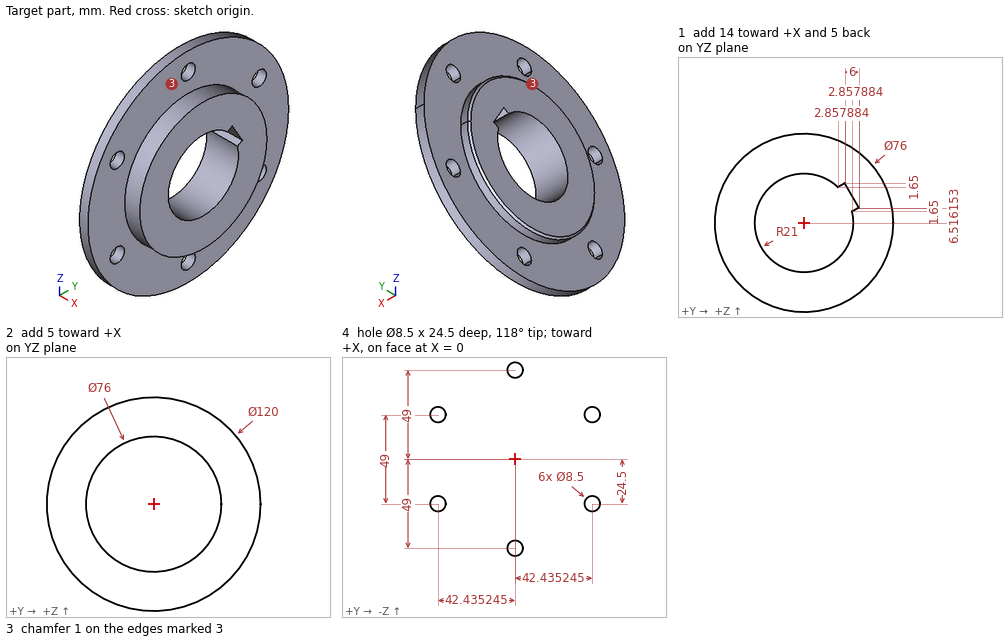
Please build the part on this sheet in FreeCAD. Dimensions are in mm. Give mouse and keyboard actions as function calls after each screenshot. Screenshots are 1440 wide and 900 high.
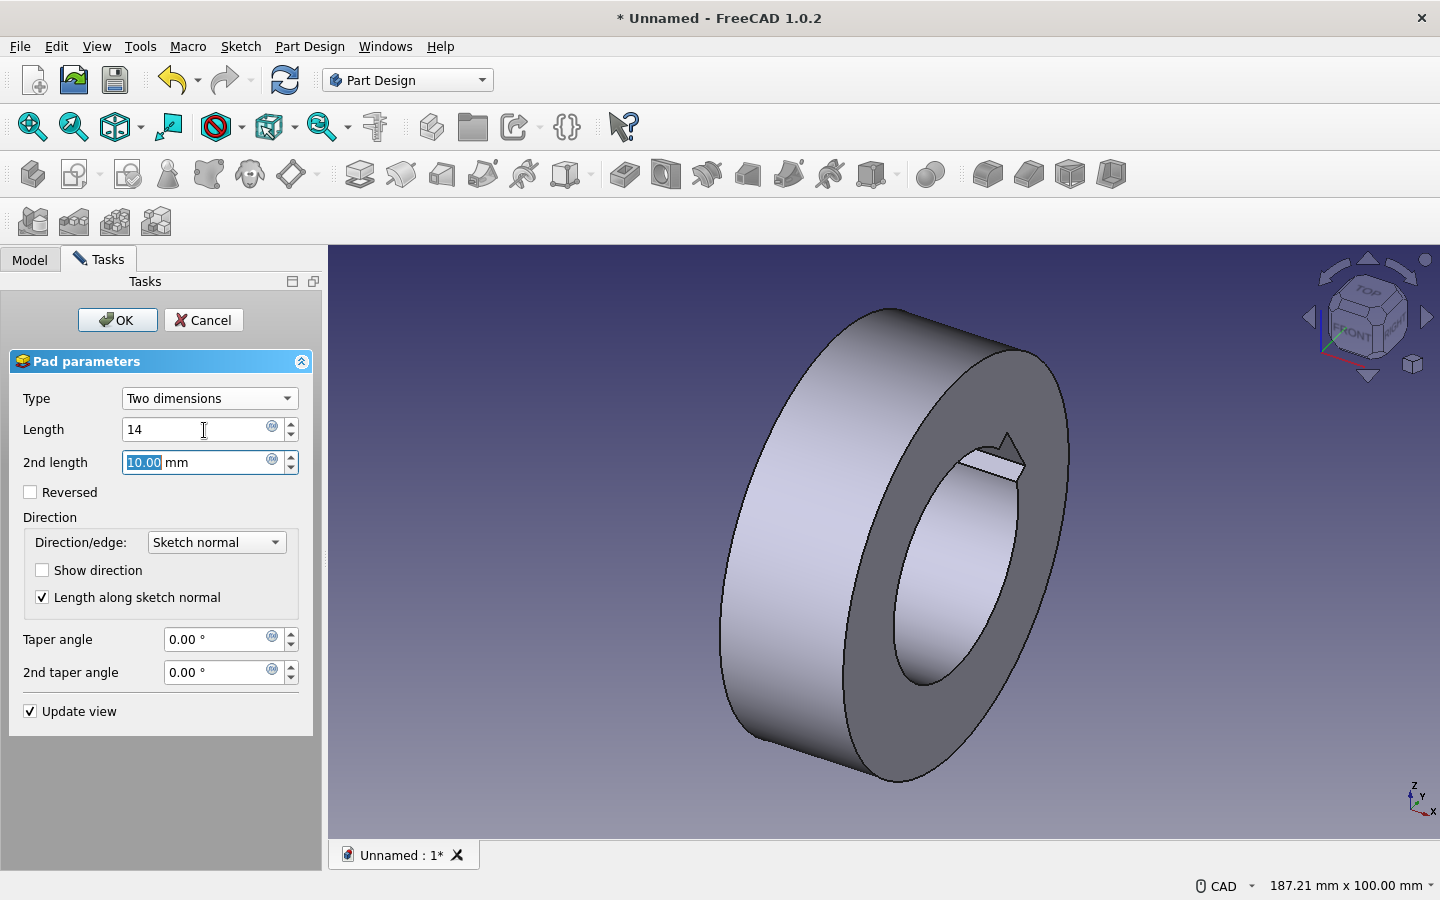
text(5)
key(Tab)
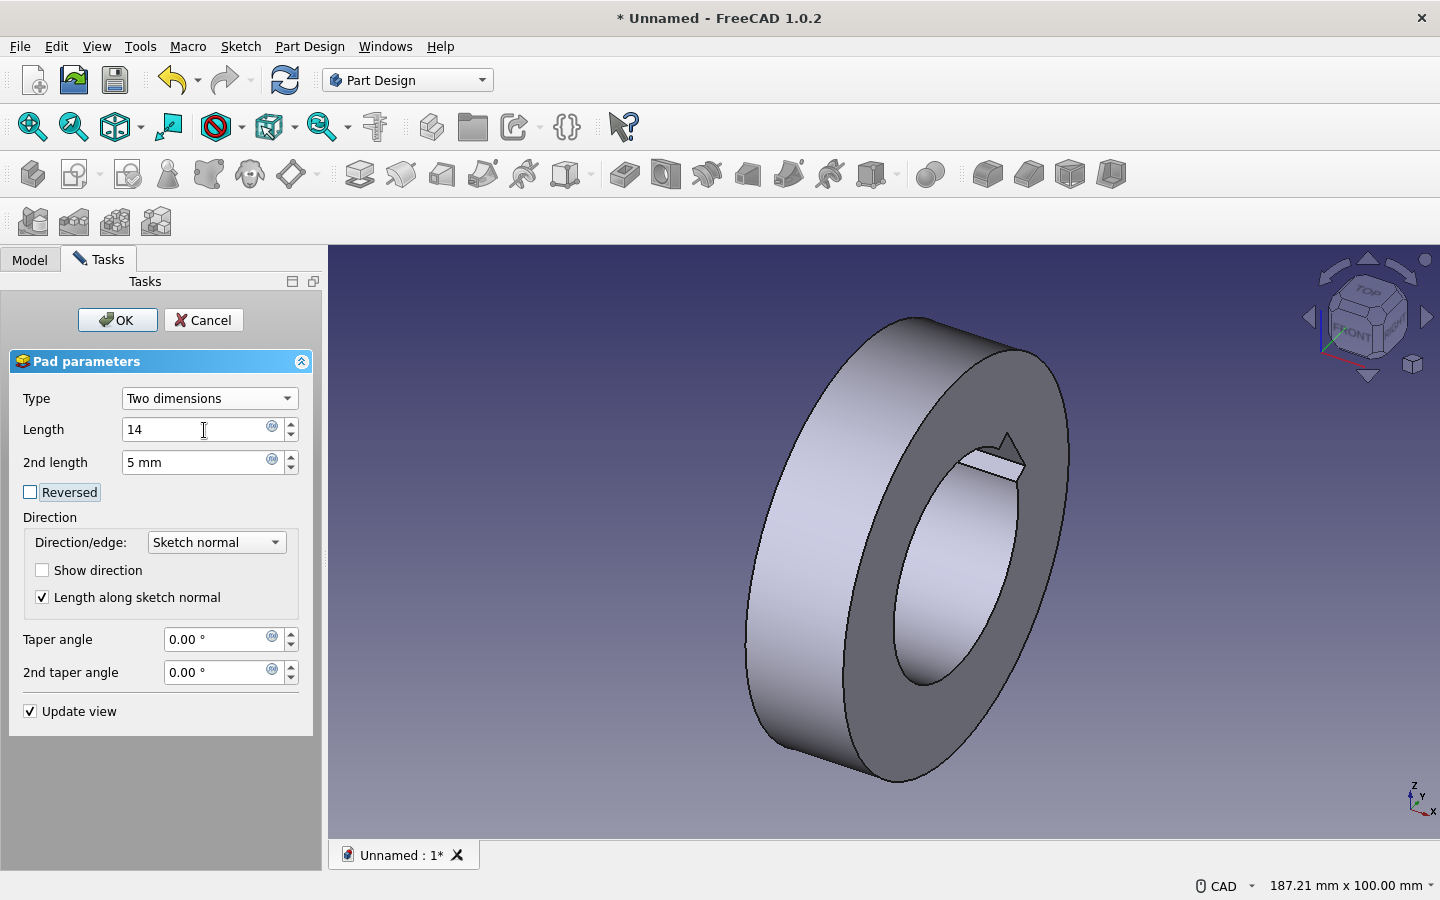
click(118, 320)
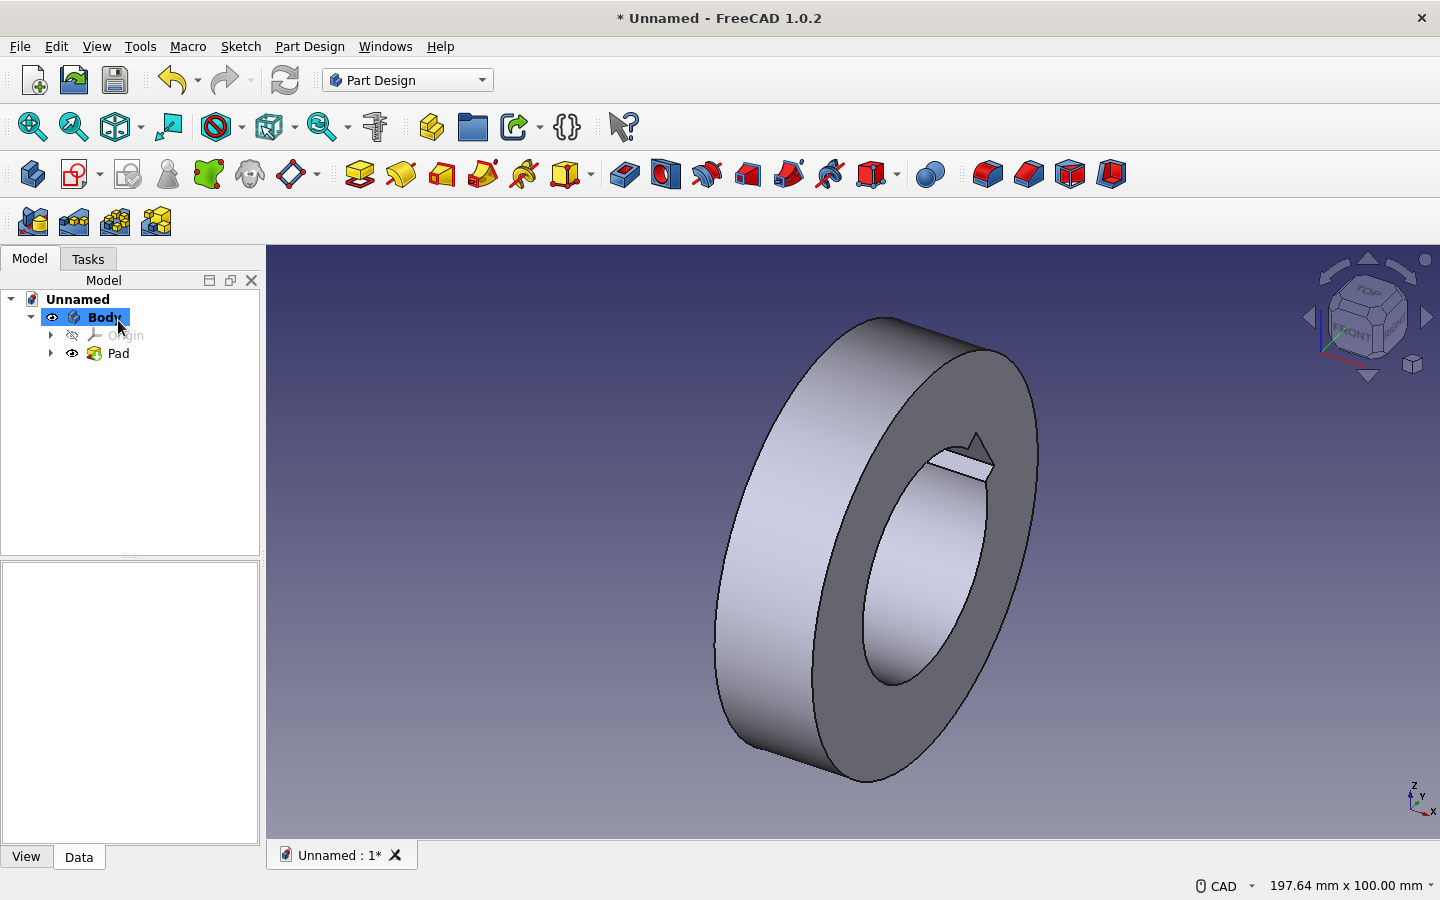
click(33, 128)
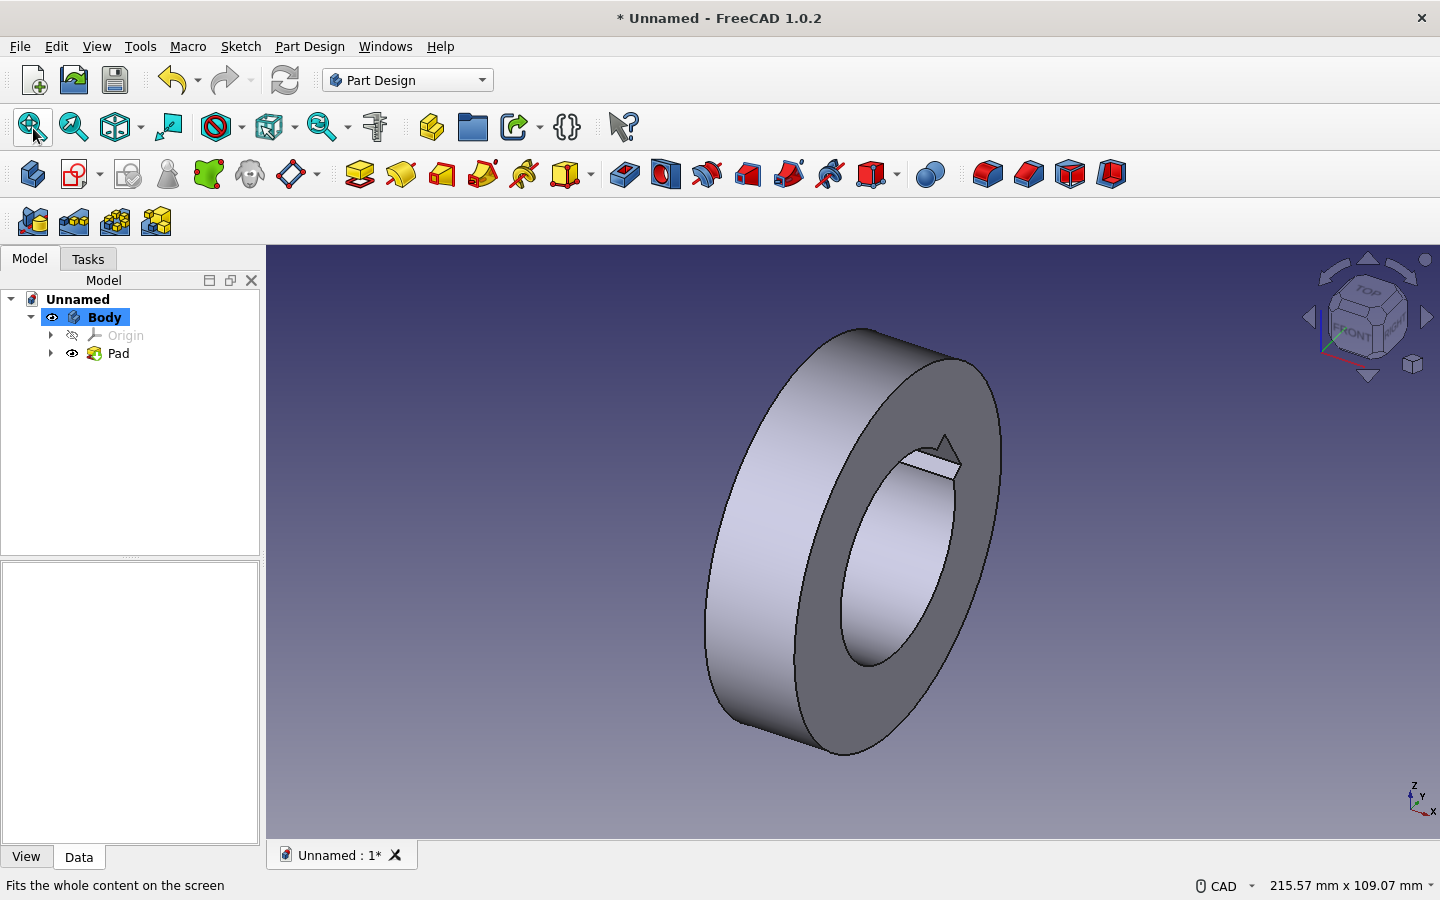
click(74, 174)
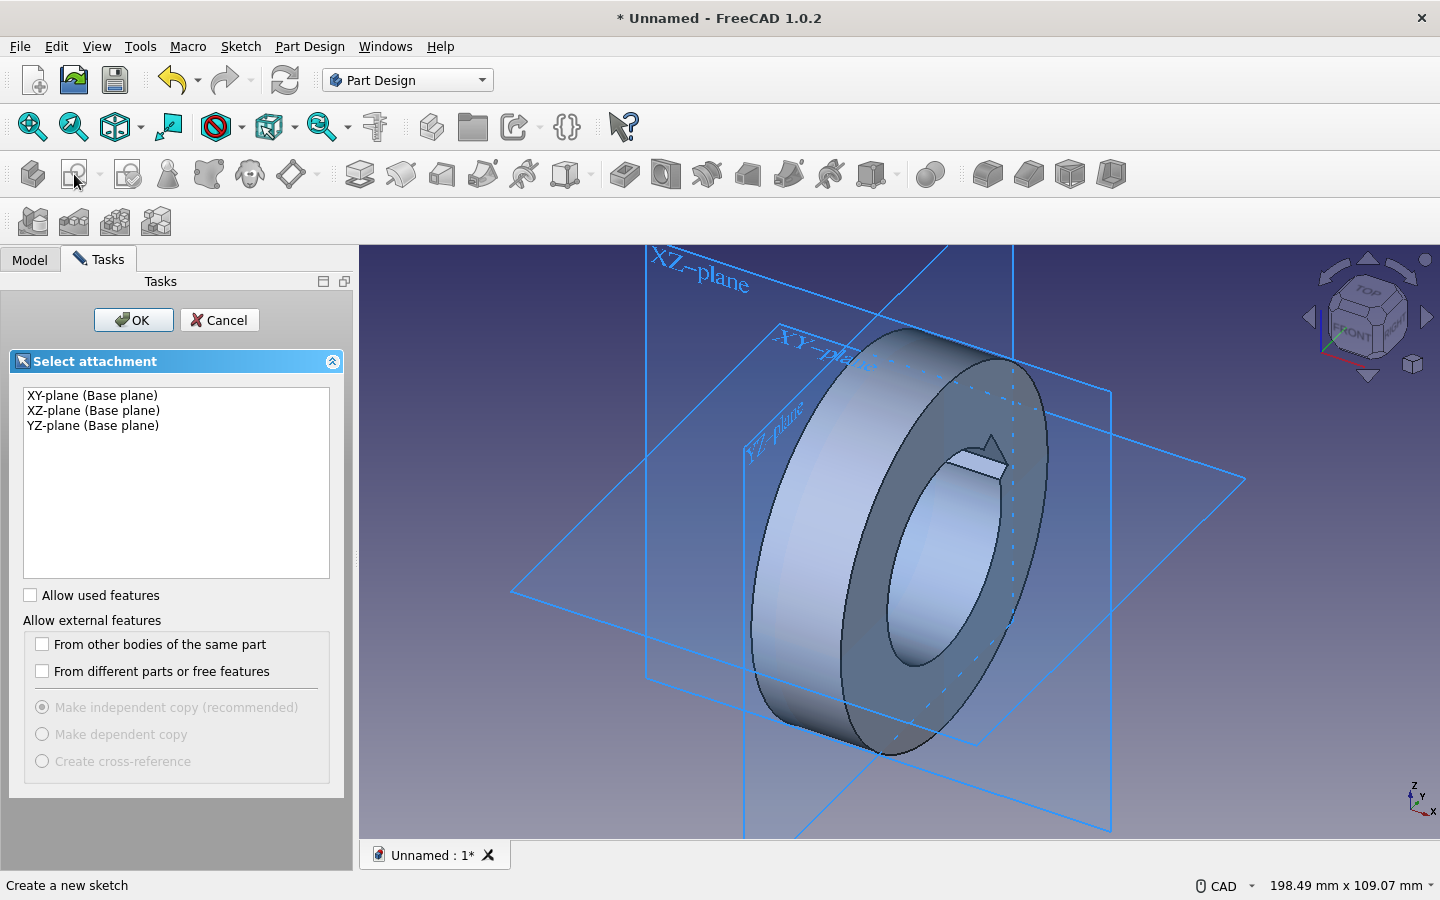
click(84, 426)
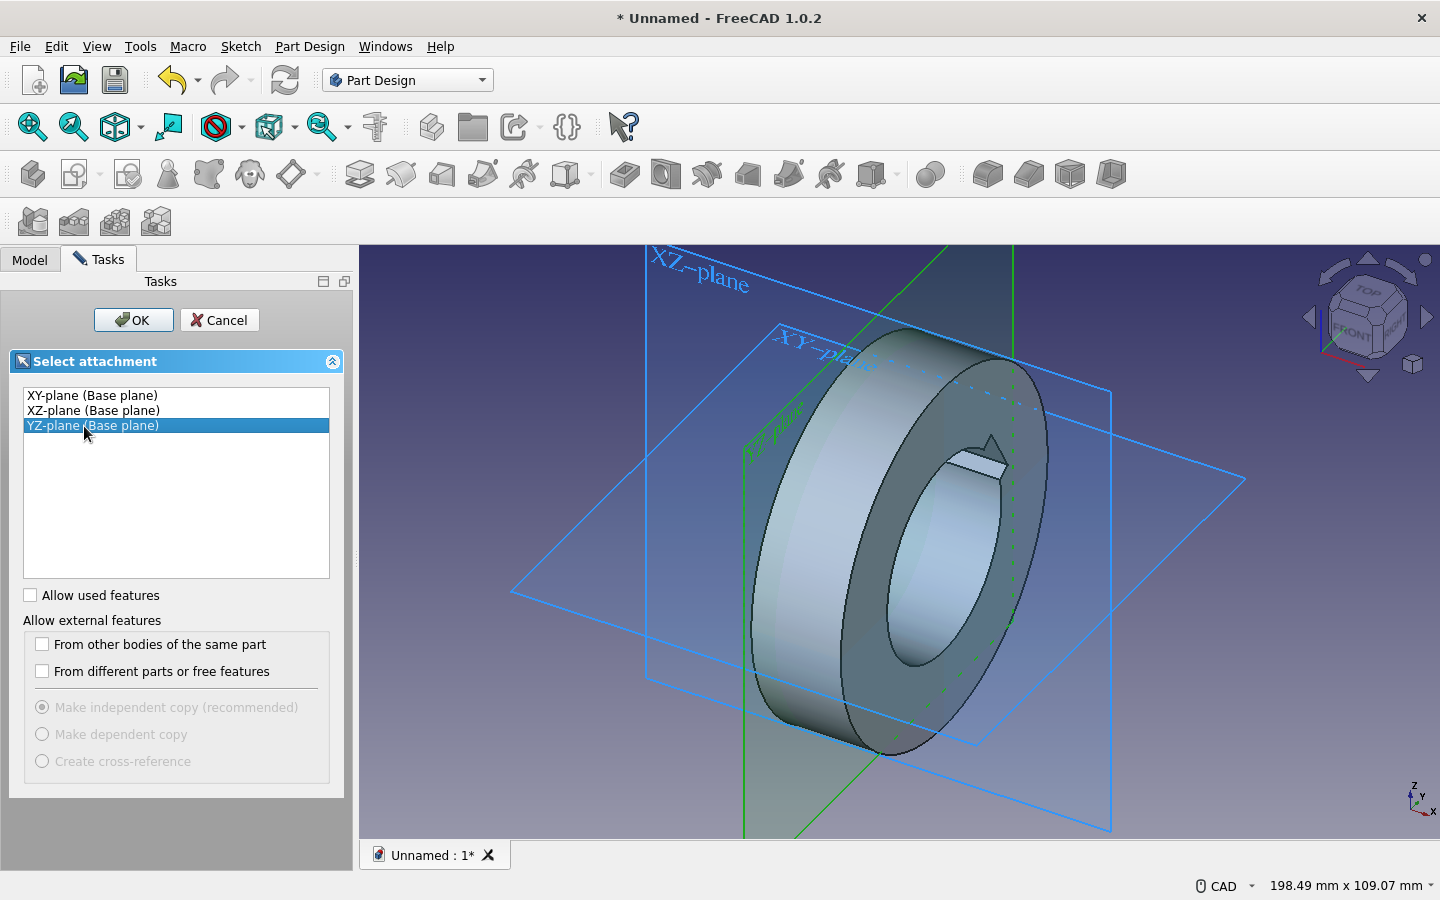
click(134, 320)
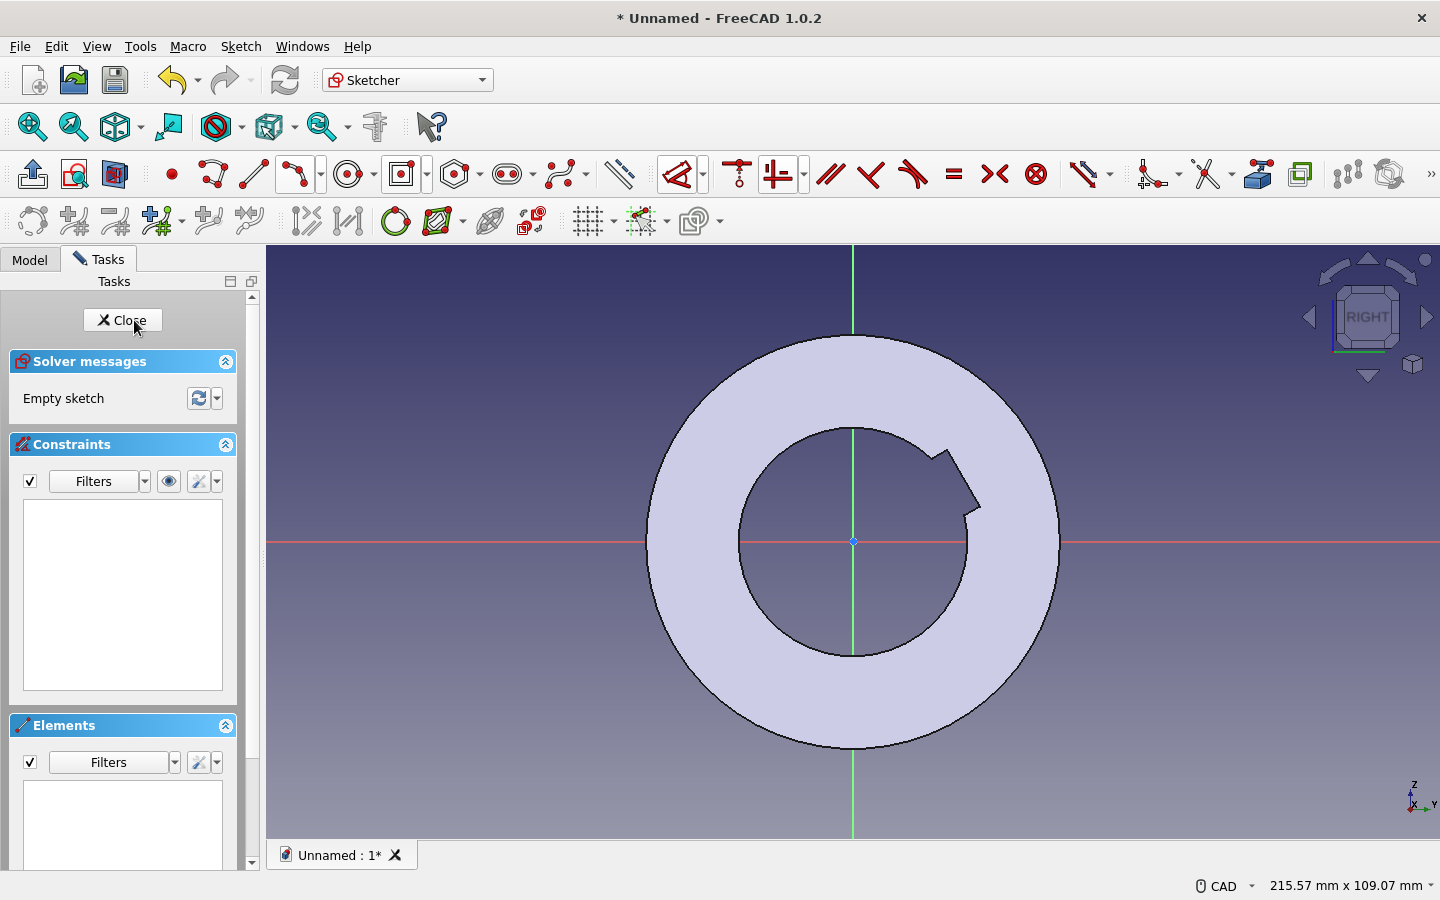
click(115, 174)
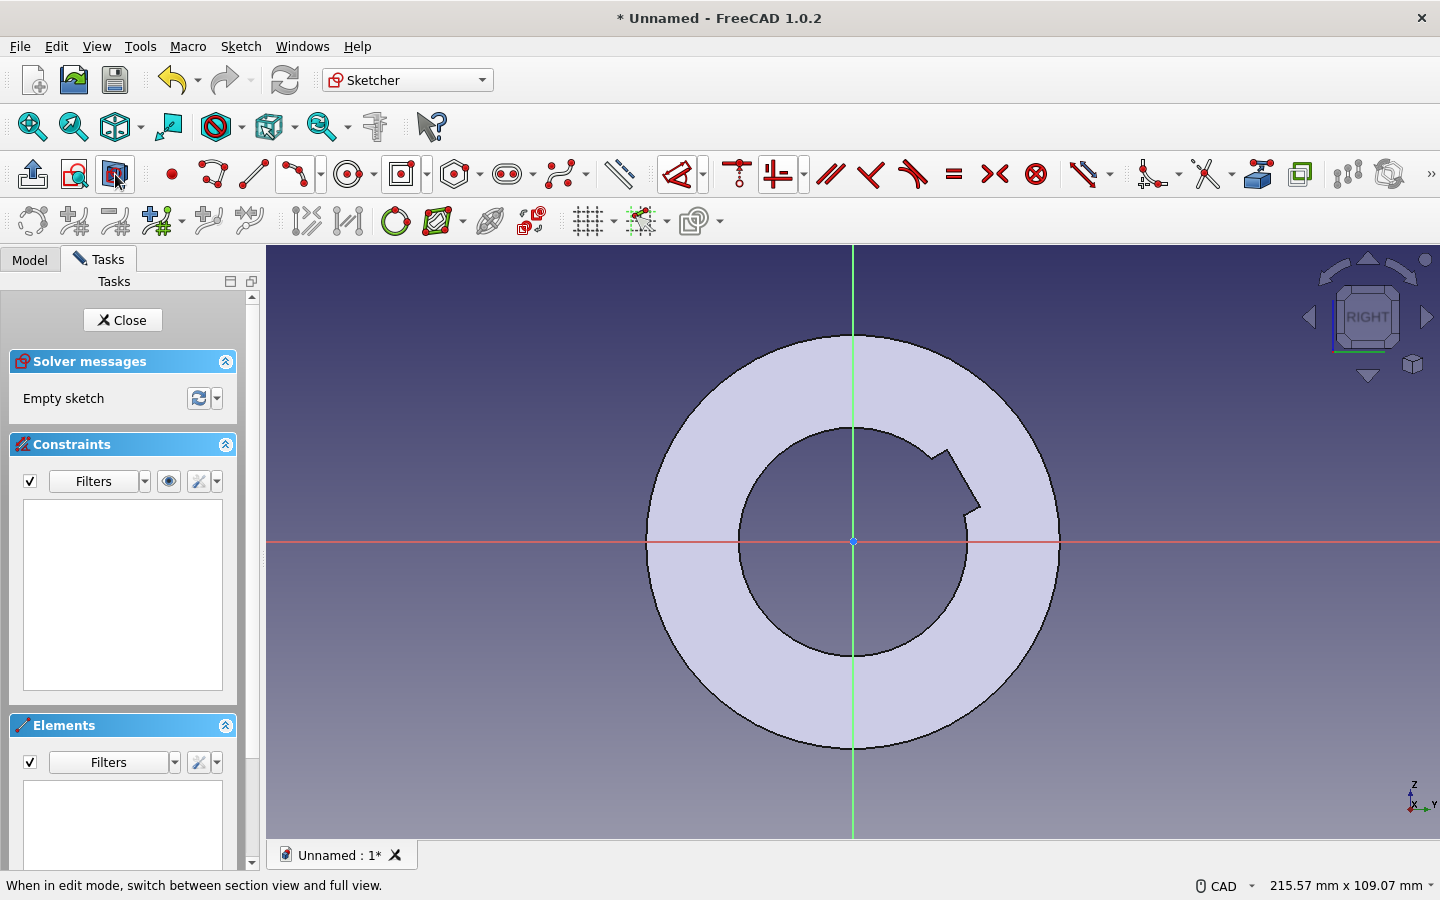
scroll(701, 542, down, 3)